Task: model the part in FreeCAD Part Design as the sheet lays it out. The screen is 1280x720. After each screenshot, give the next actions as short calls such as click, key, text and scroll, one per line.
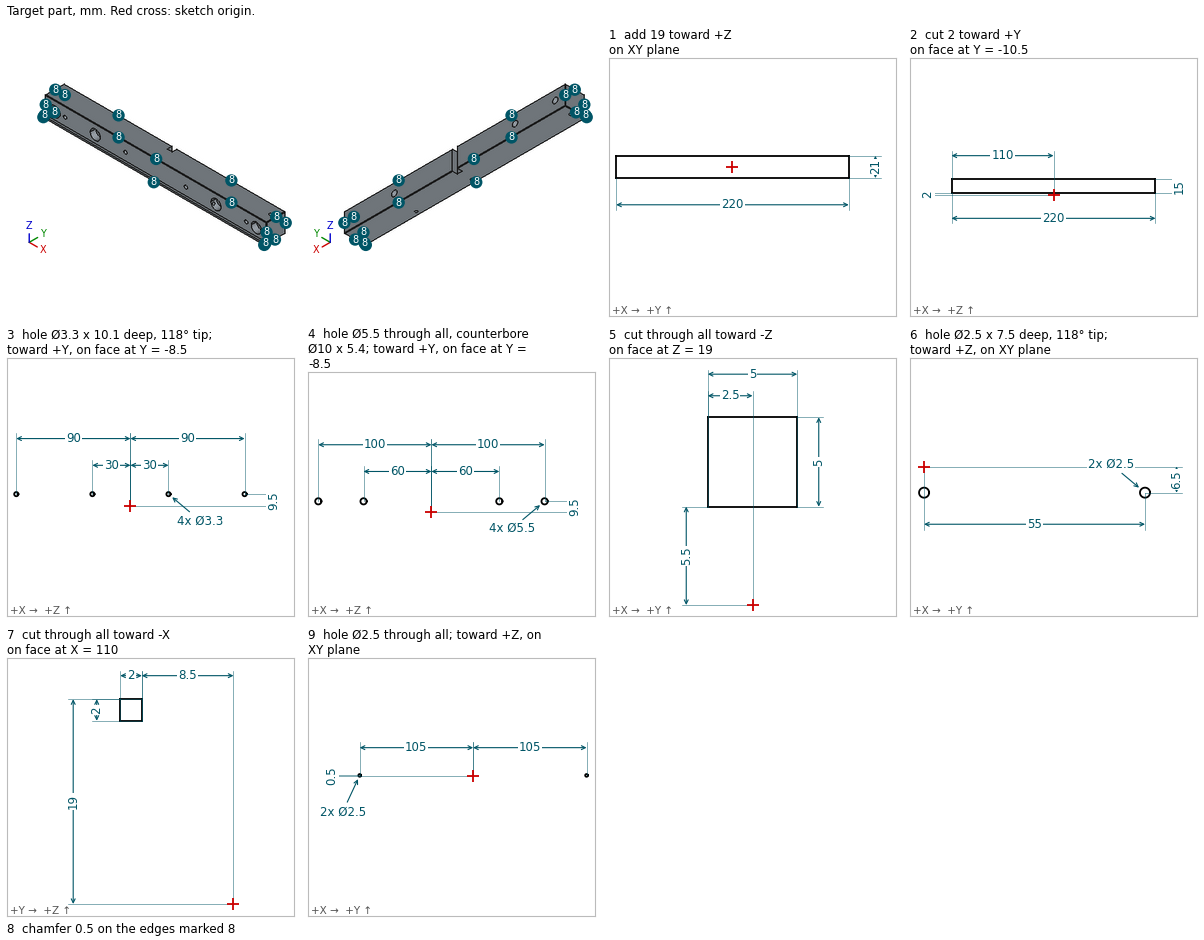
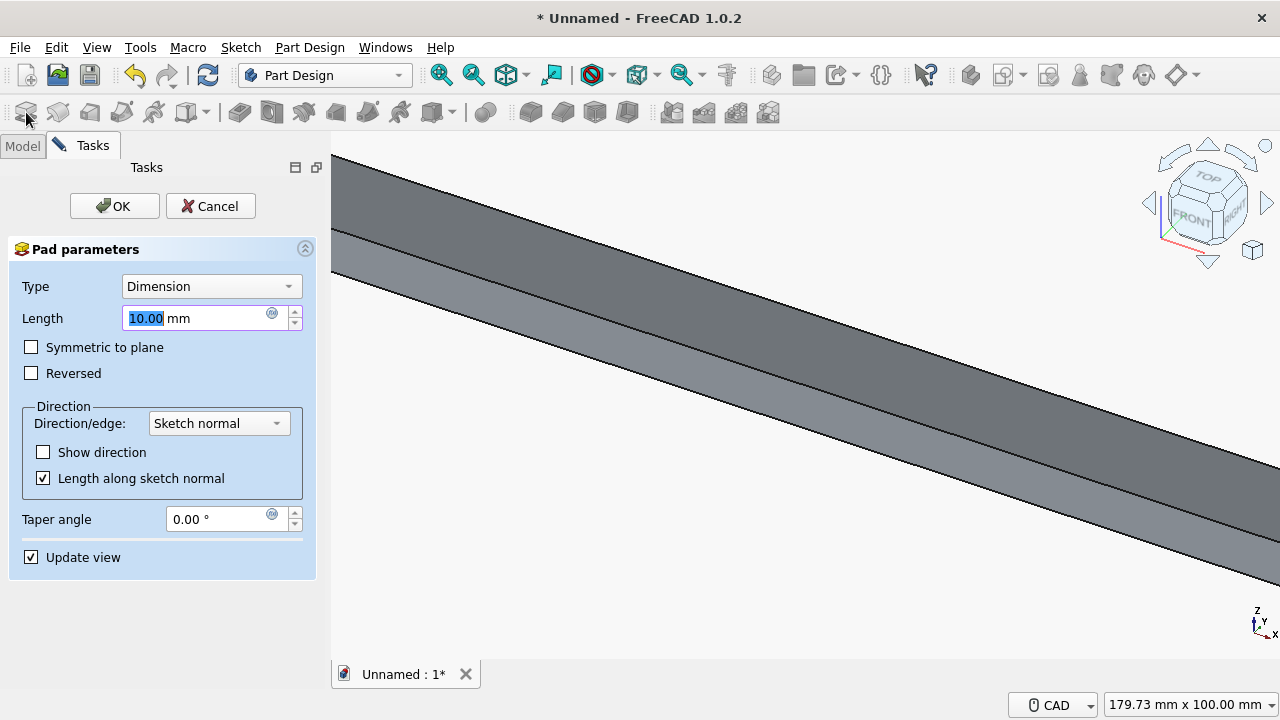
text(19)
key(Tab)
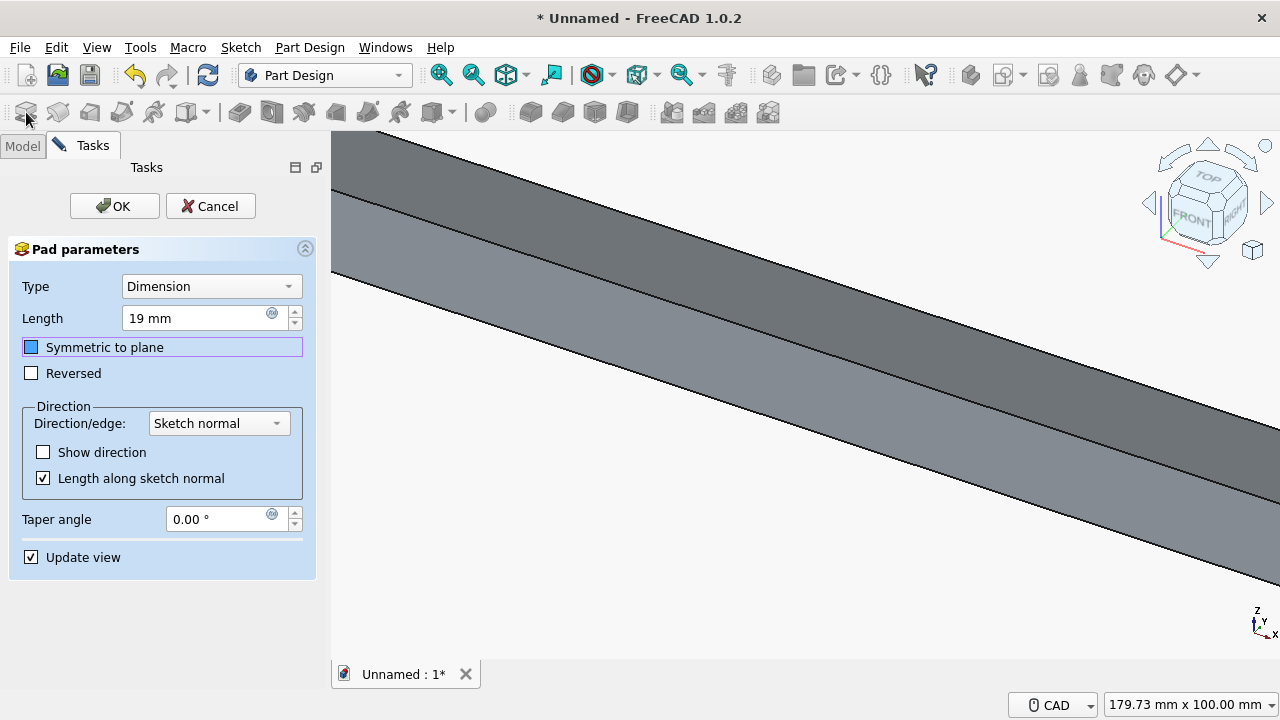
click(115, 206)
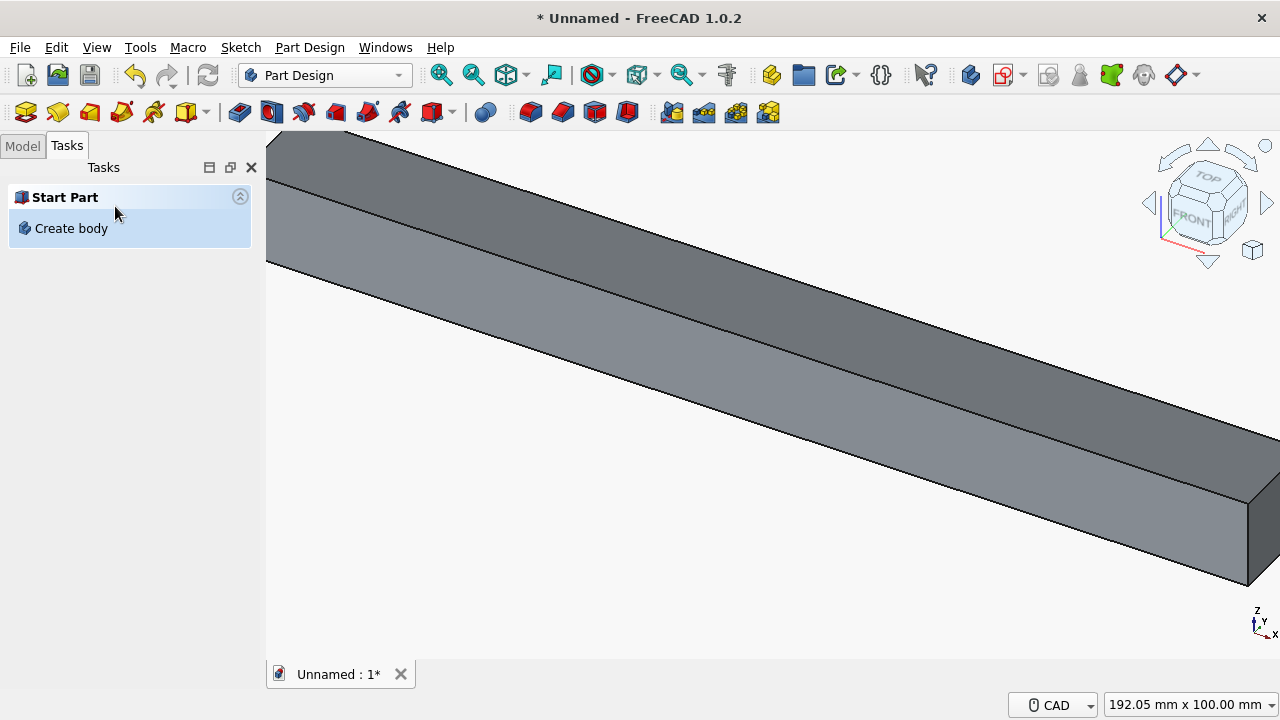
click(442, 76)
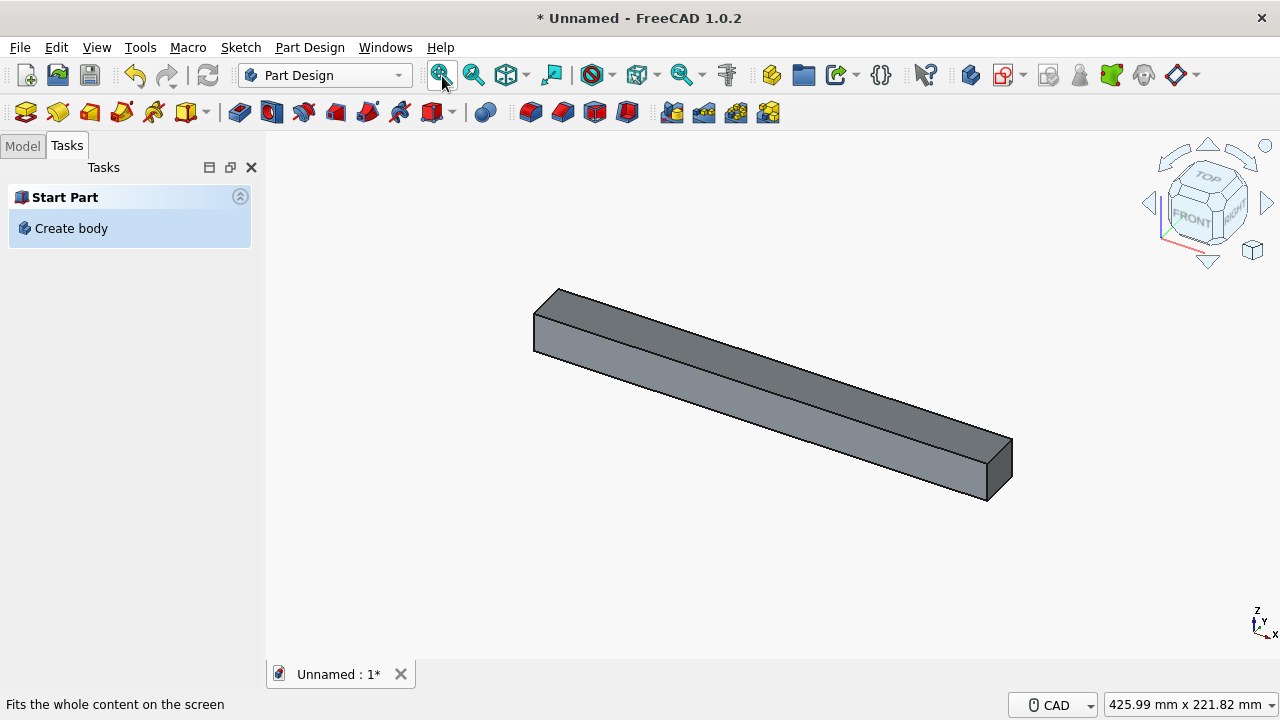
click(955, 471)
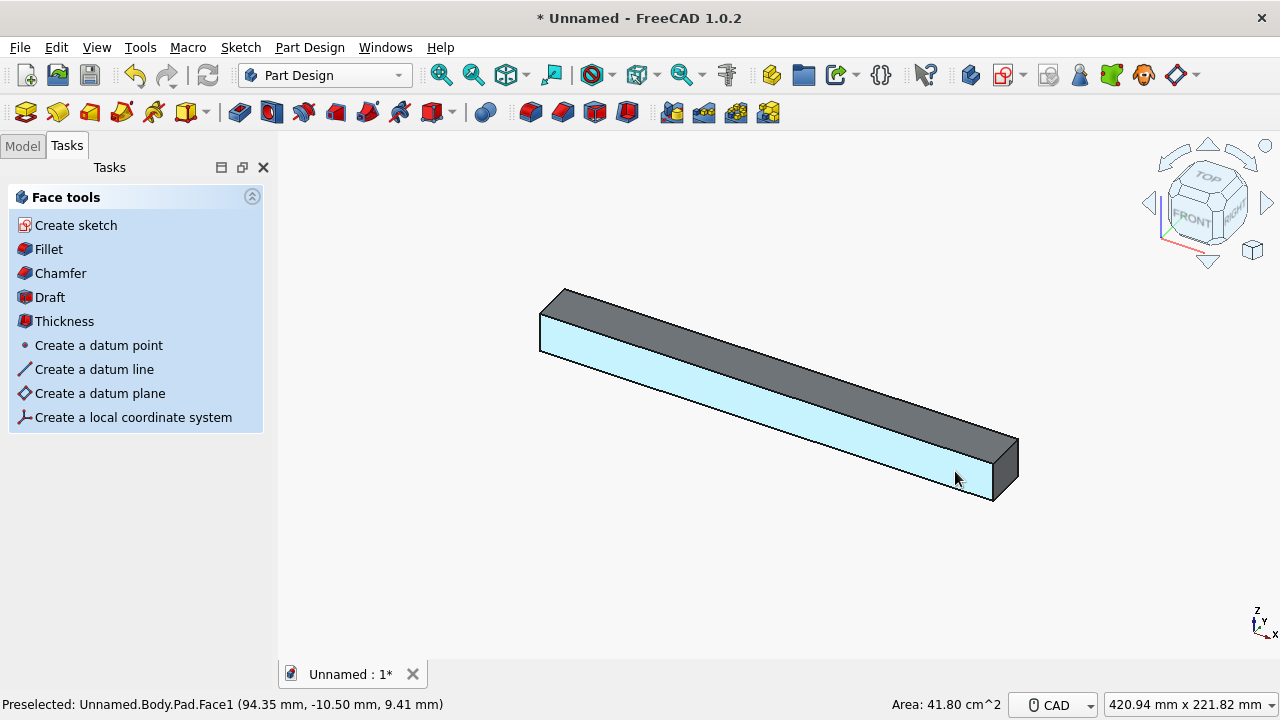
click(1004, 76)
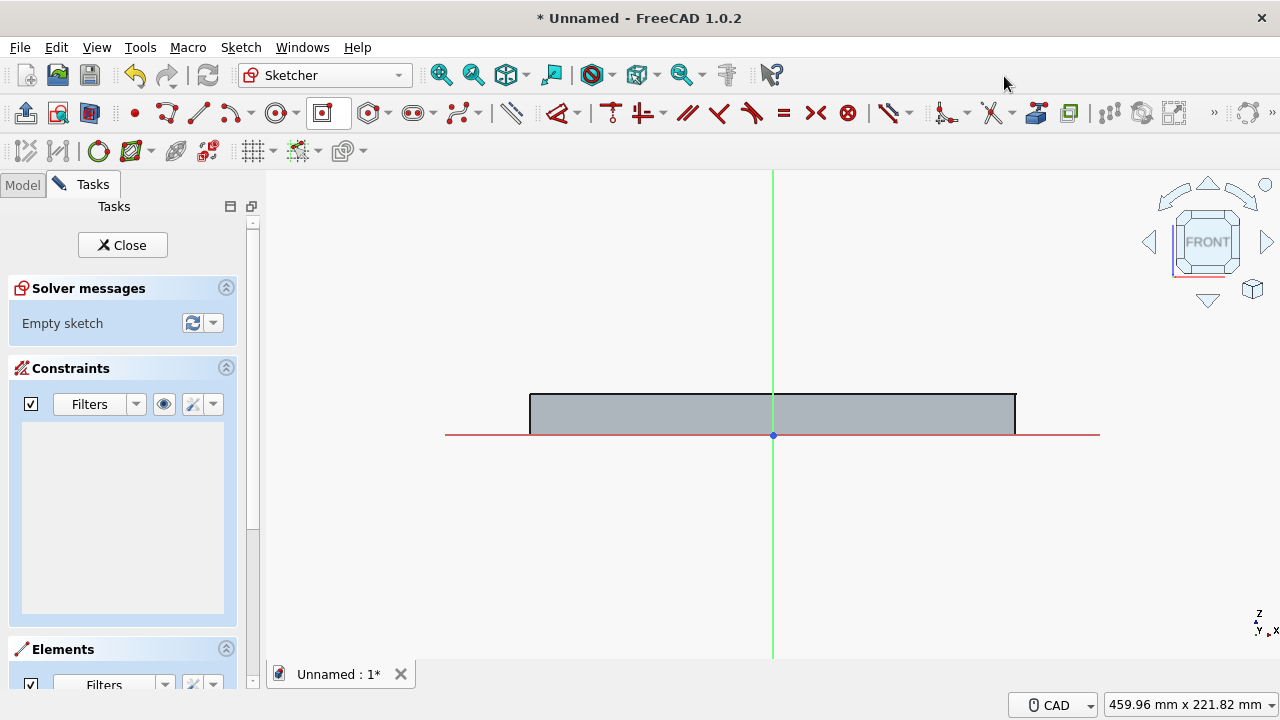
click(346, 114)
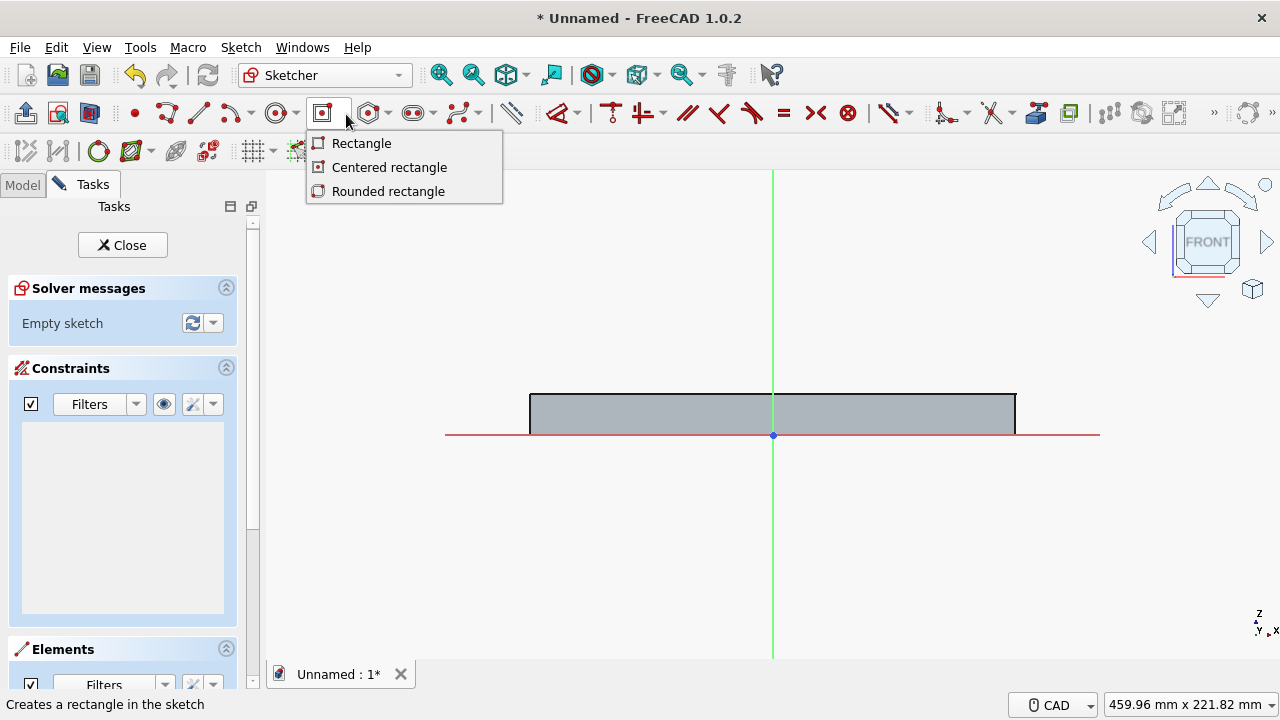
click(404, 143)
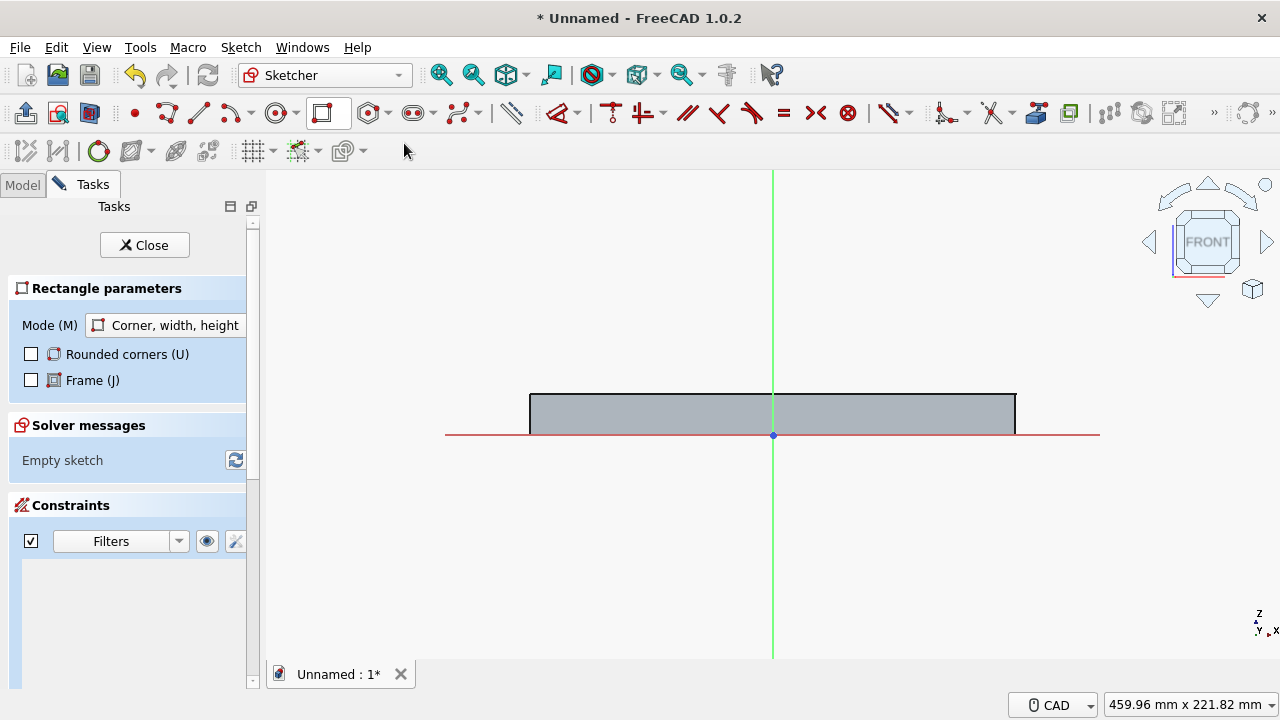
click(531, 398)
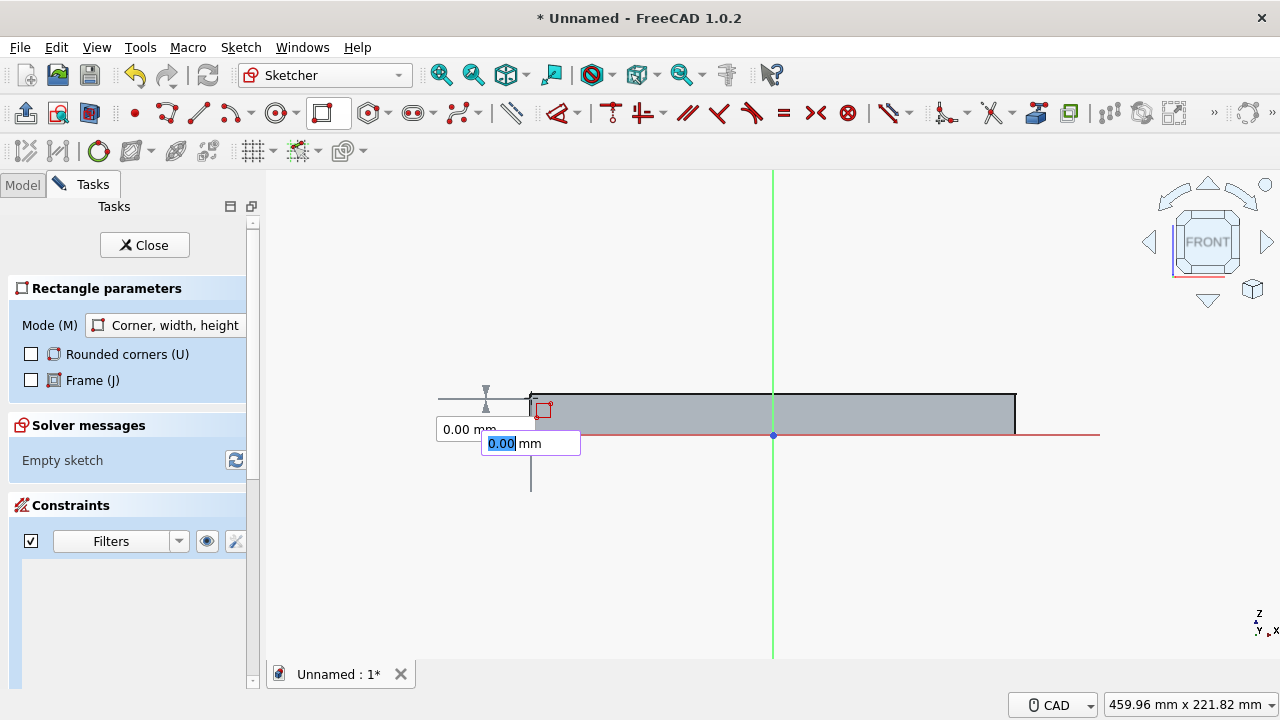
scroll(1015, 431, up, 7)
move(1015, 430)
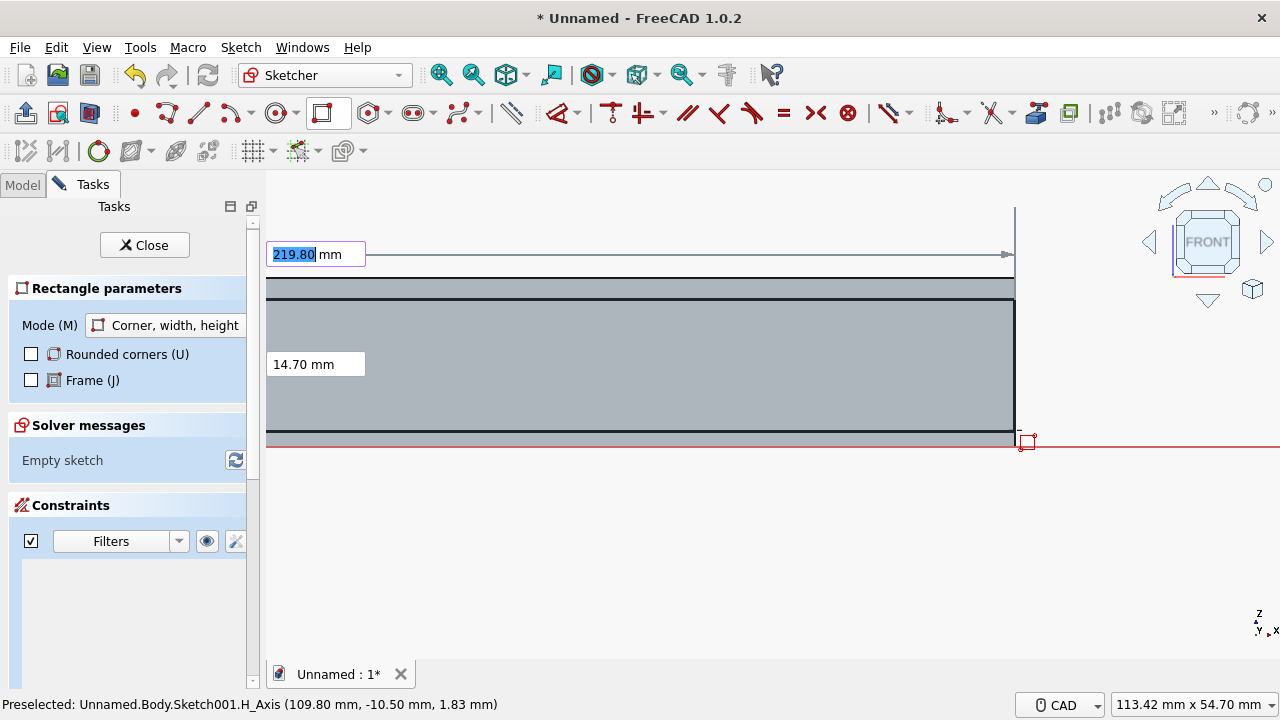
text(220)
key(Tab)
text(15)
key(Return)
key(Escape)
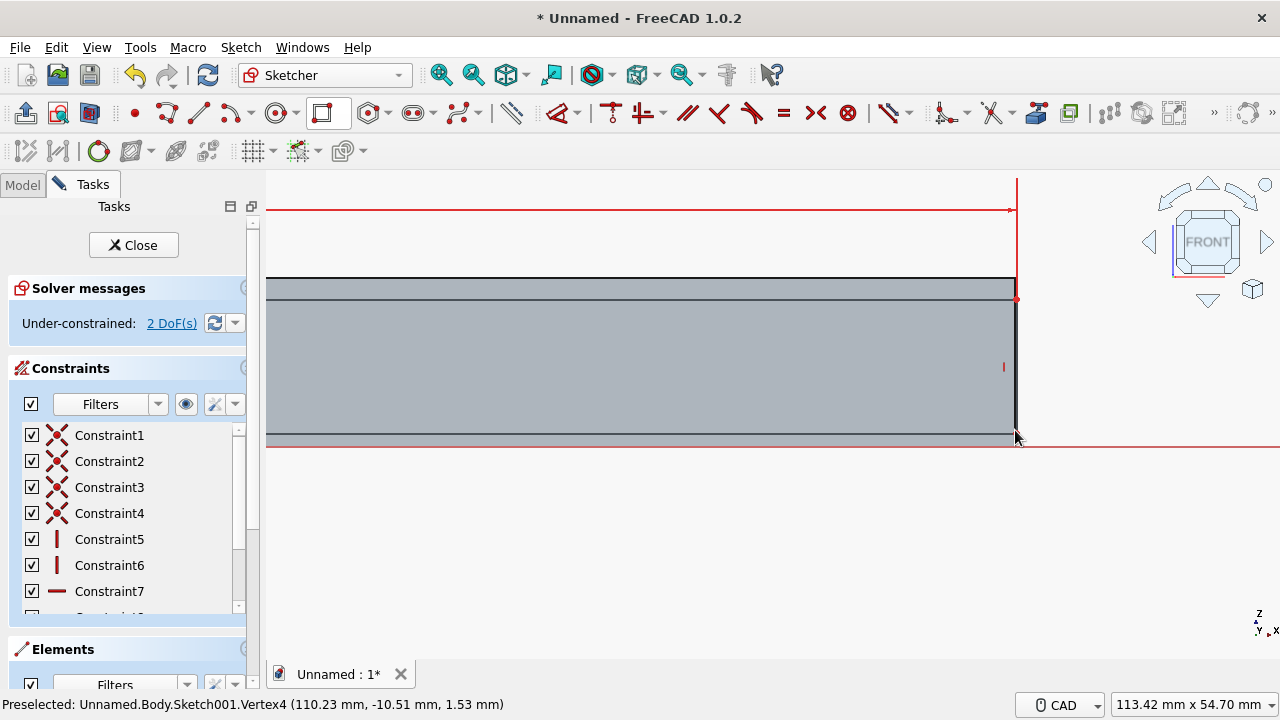
click(558, 114)